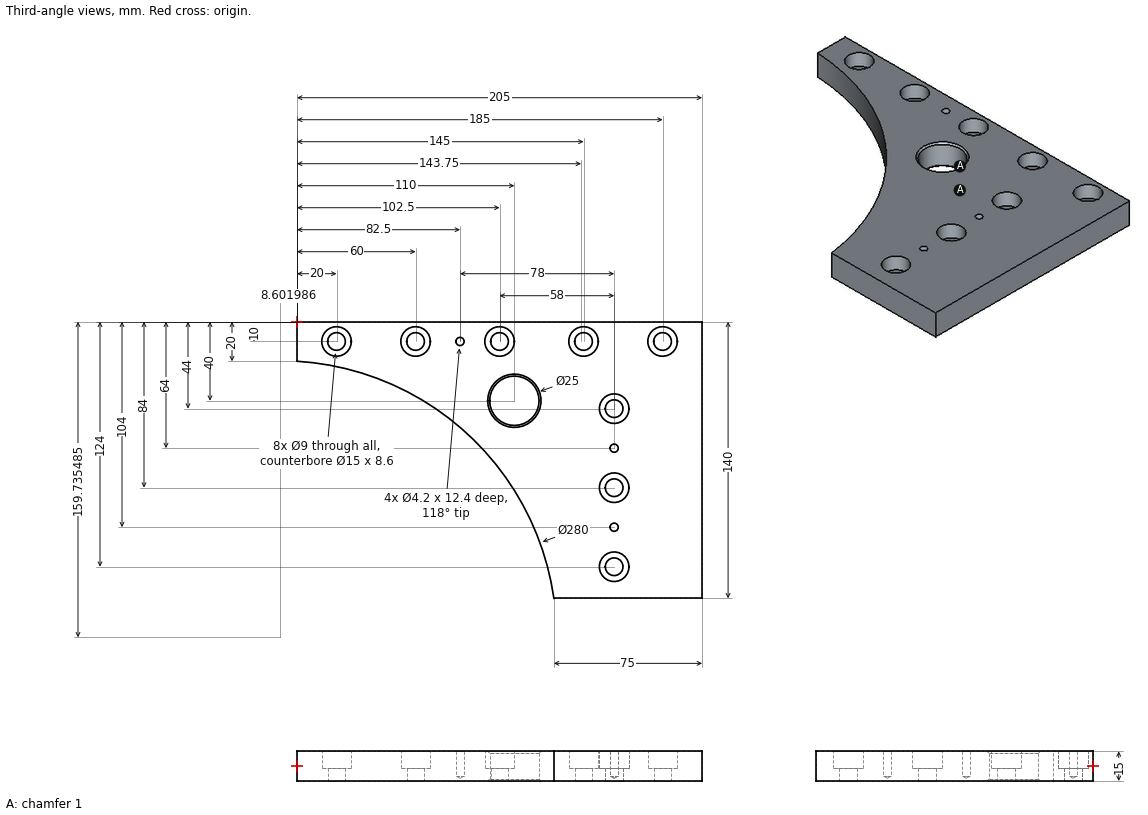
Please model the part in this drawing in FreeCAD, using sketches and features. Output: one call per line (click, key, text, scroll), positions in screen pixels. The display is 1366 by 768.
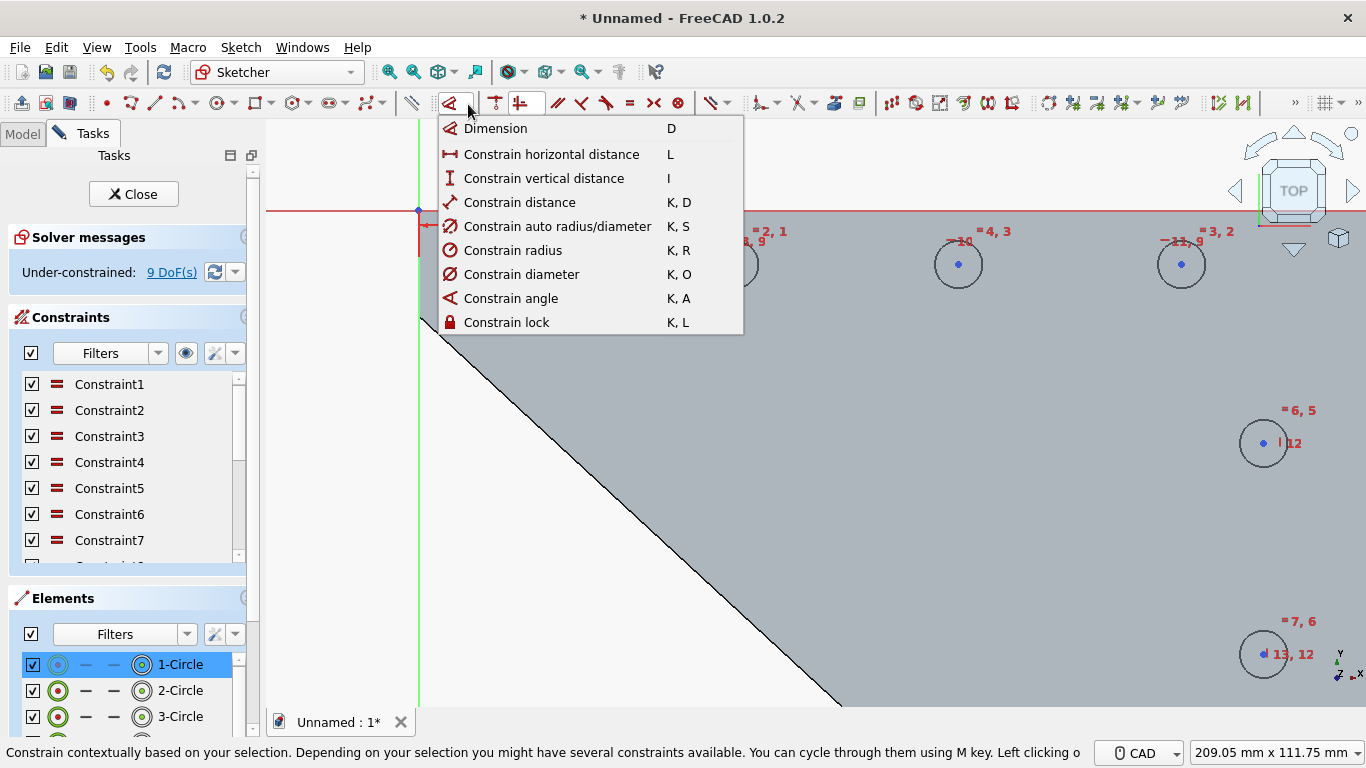
click(591, 178)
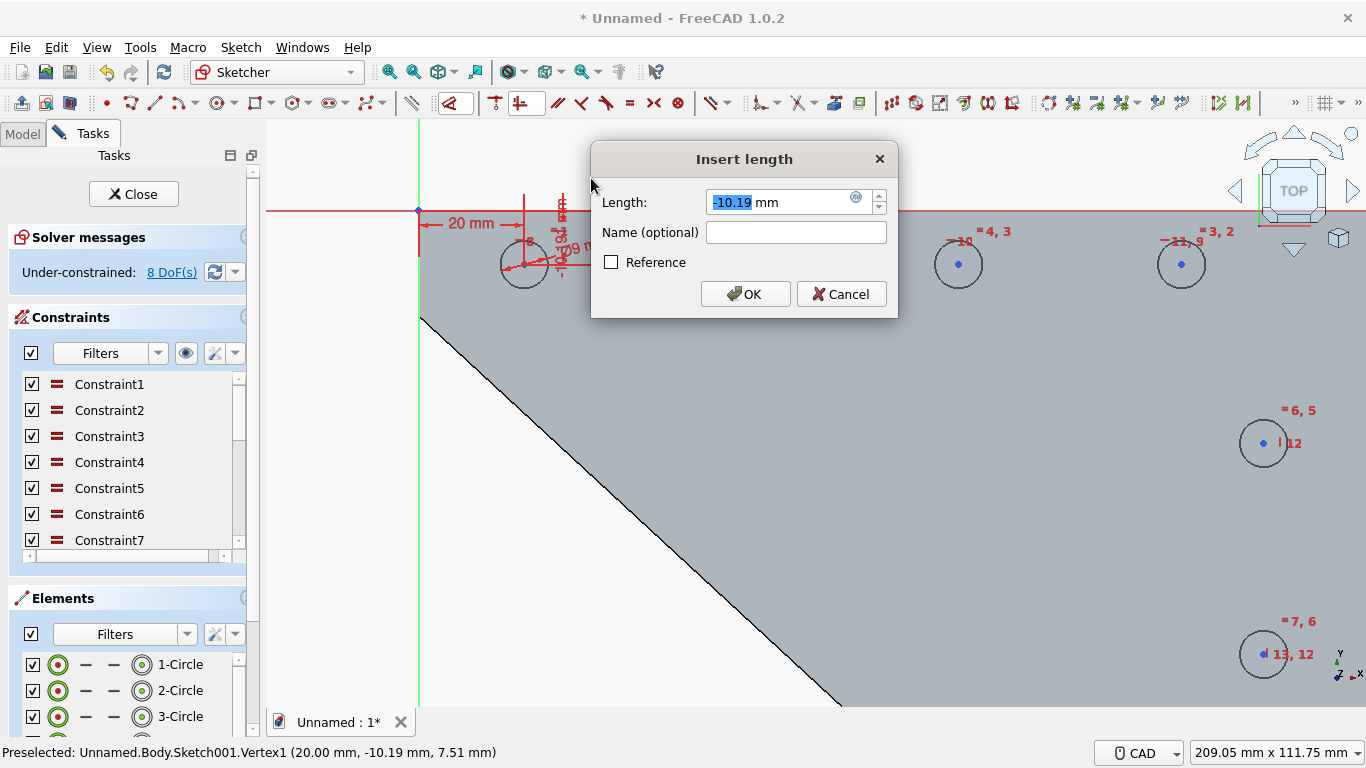
text(-10)
key(Return)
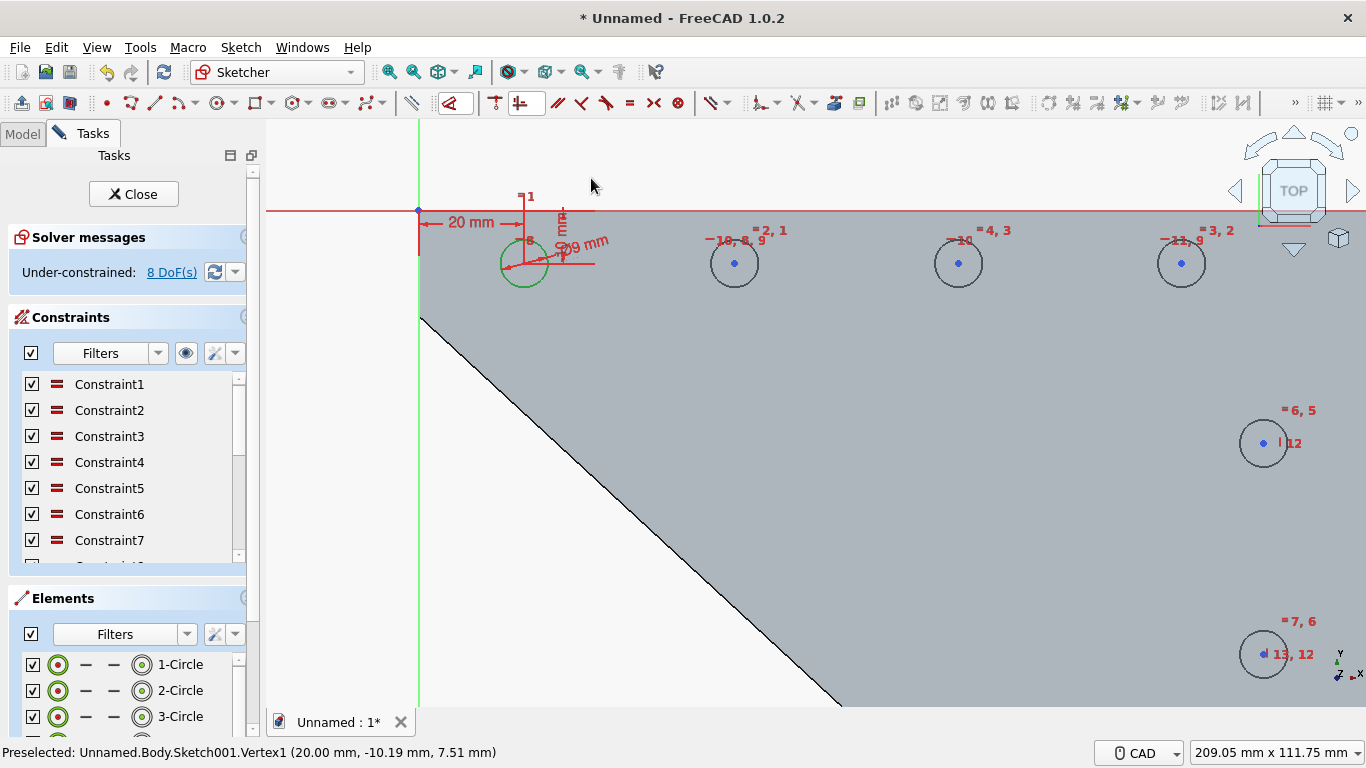
click(735, 264)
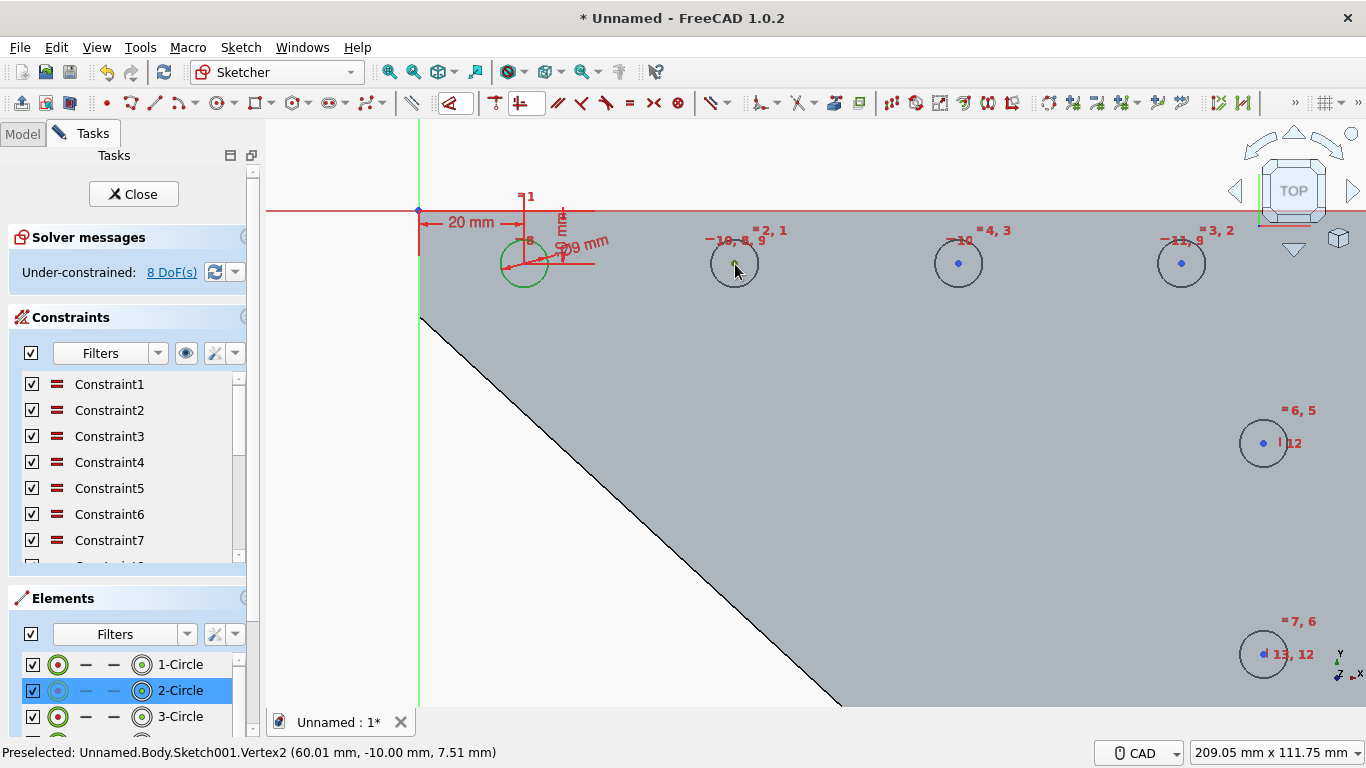
key(l)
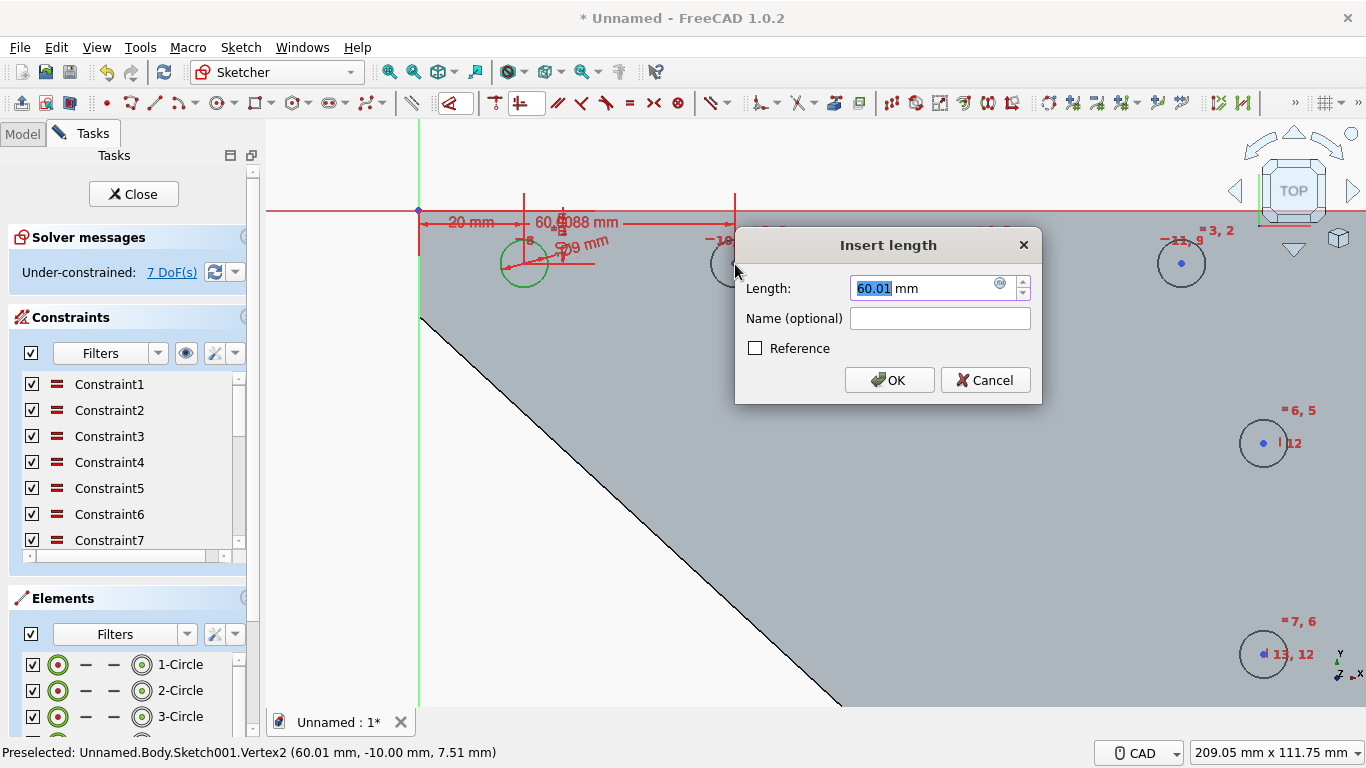
text(60)
key(Return)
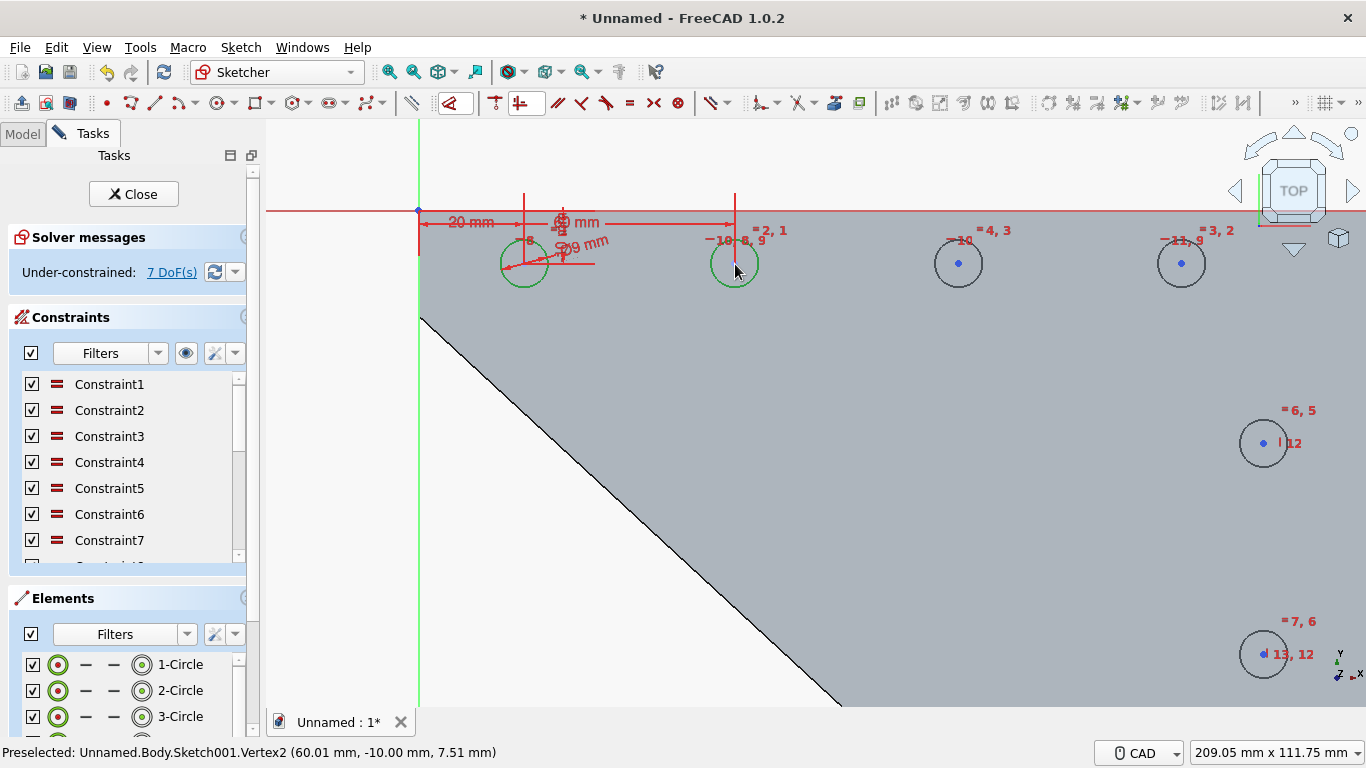
scroll(541, 248, down, 3)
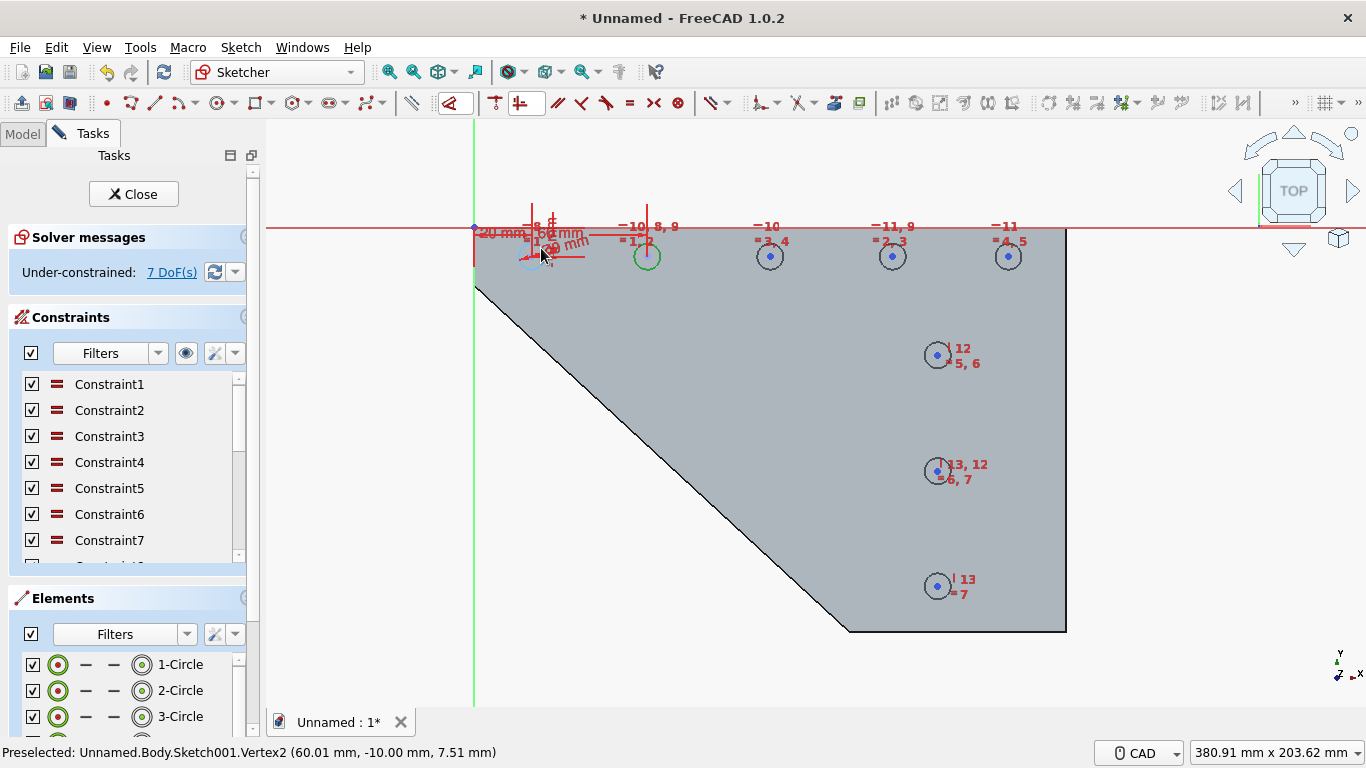
click(938, 355)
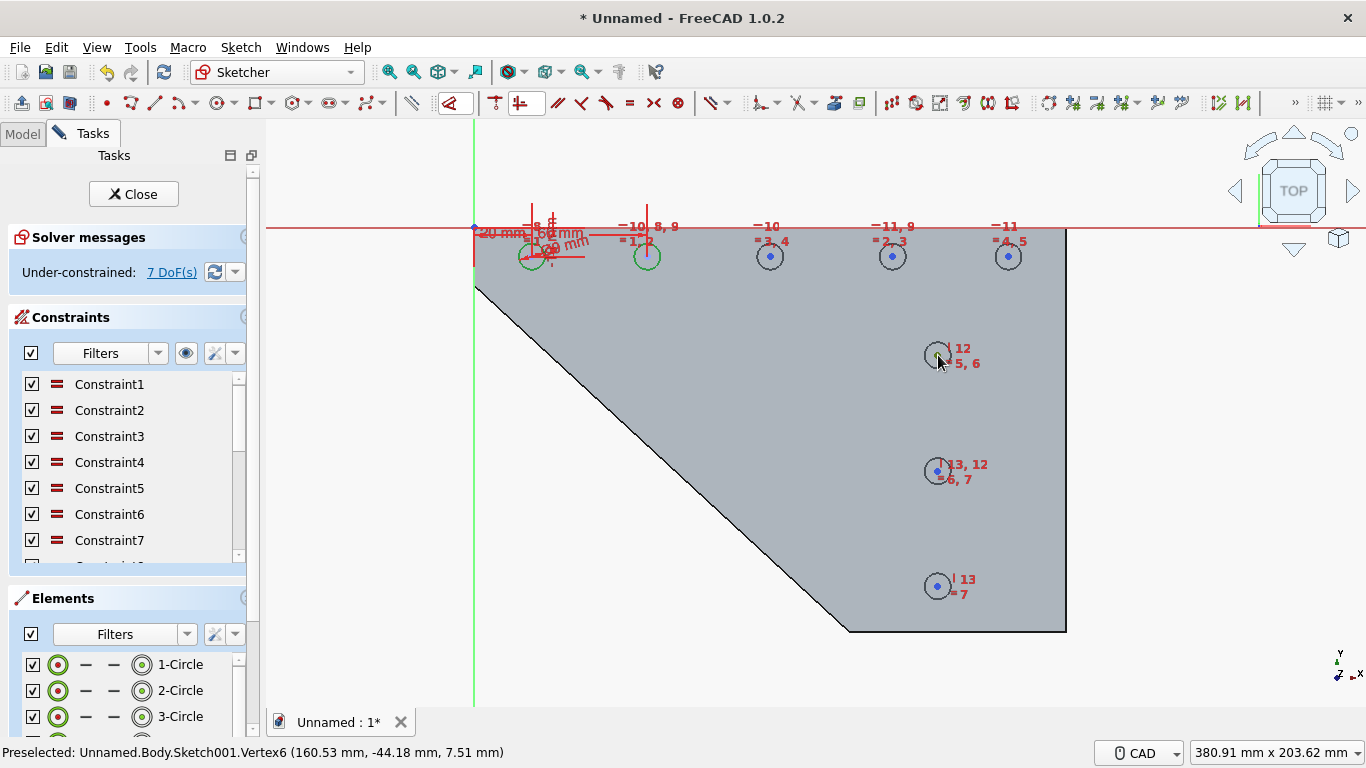
click(468, 104)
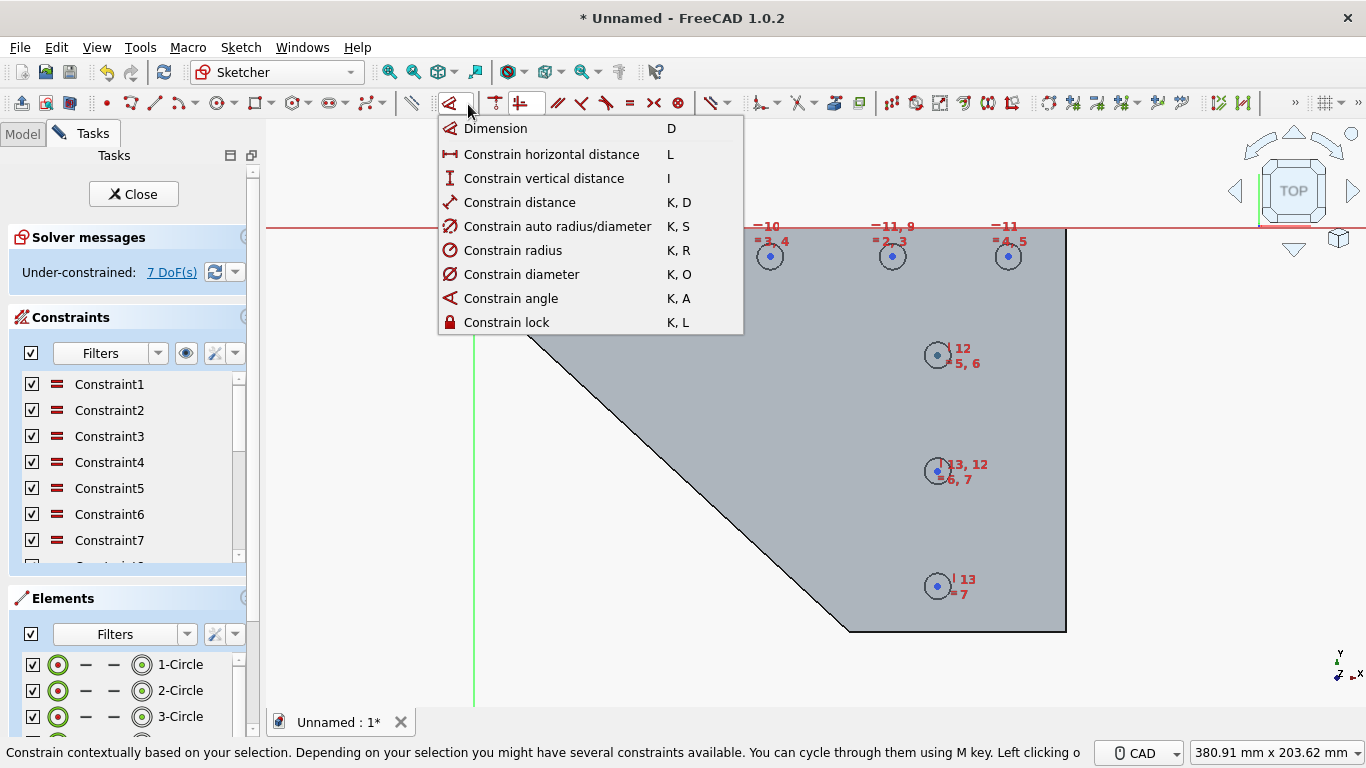
click(591, 178)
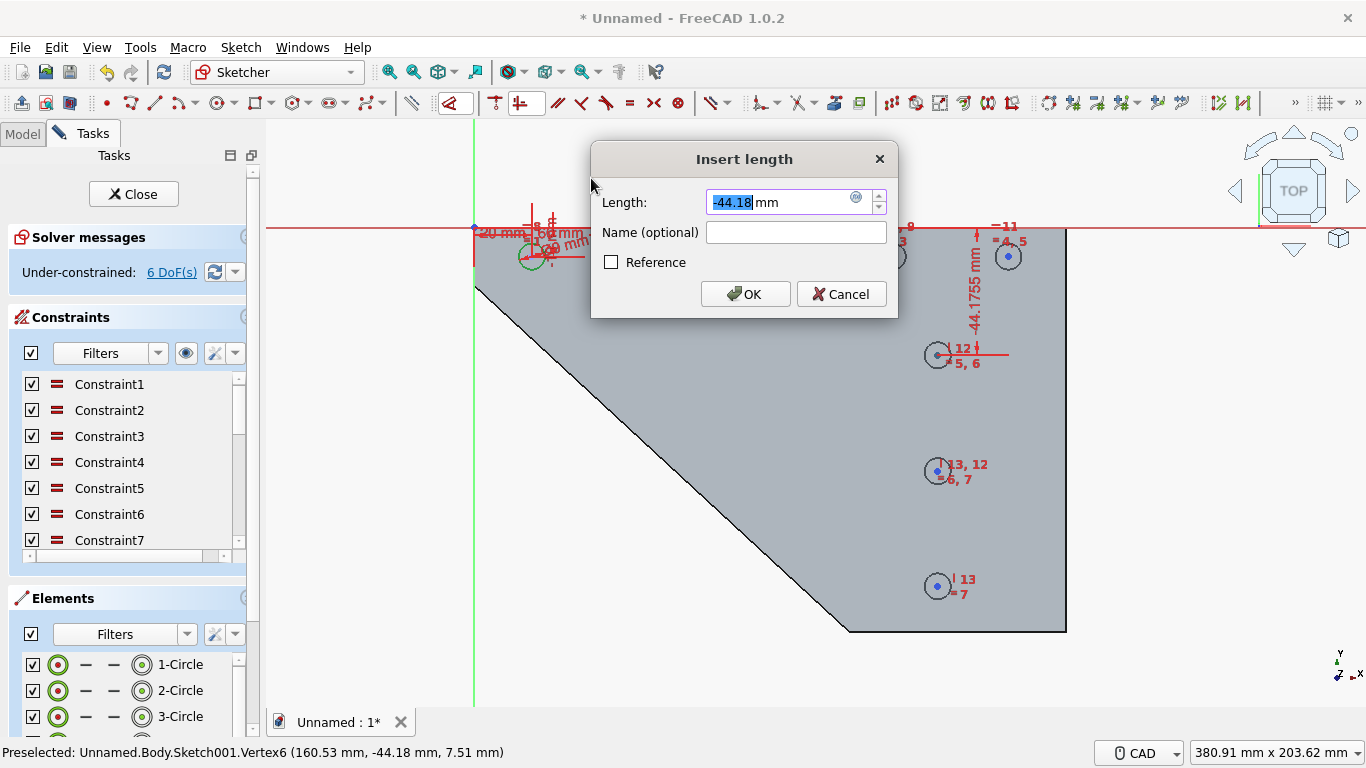
text(-44)
key(Return)